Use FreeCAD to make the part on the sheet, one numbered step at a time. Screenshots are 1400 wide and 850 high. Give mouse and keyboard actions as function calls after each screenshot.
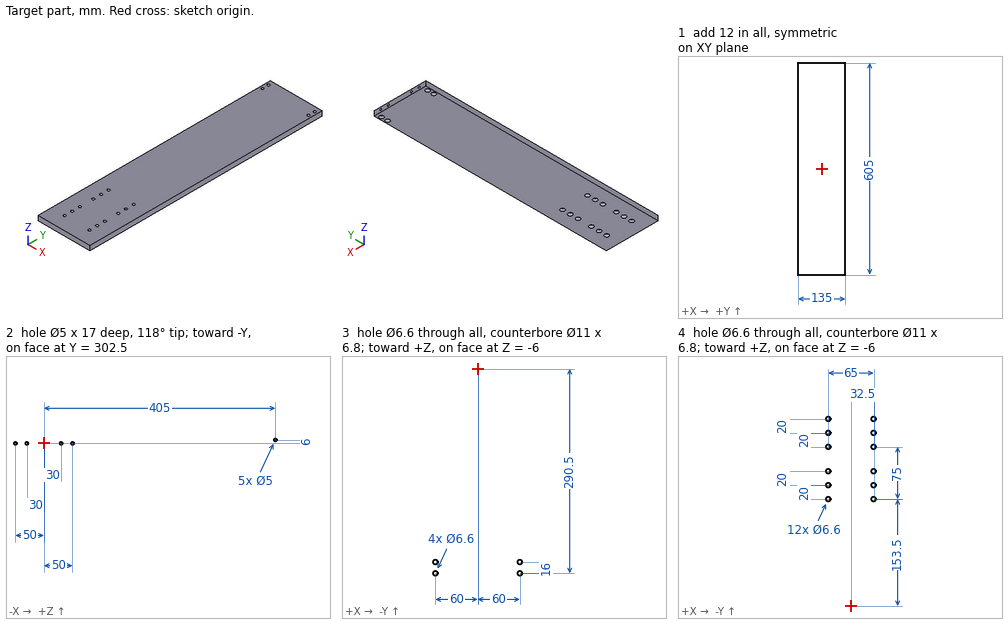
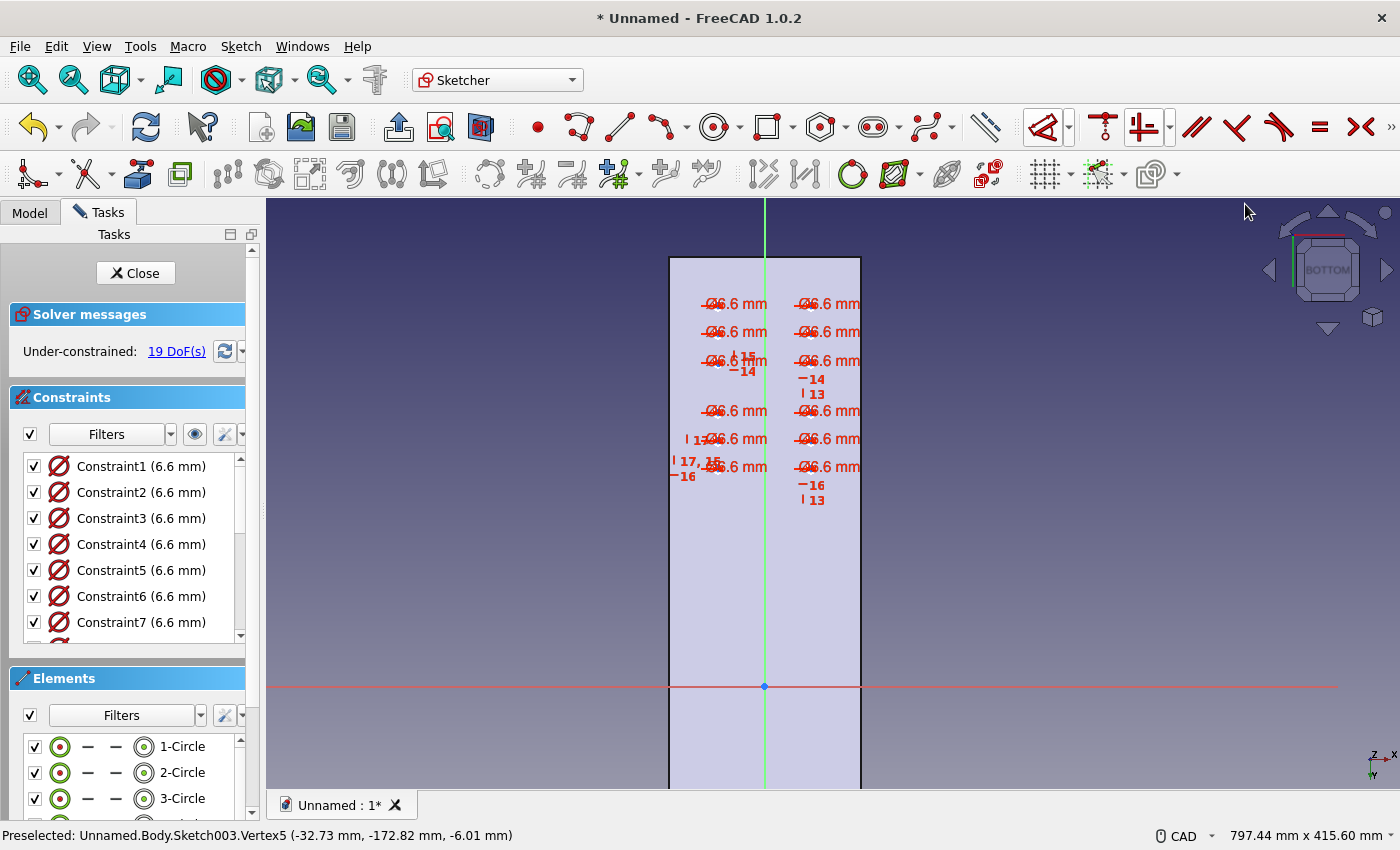
click(718, 363)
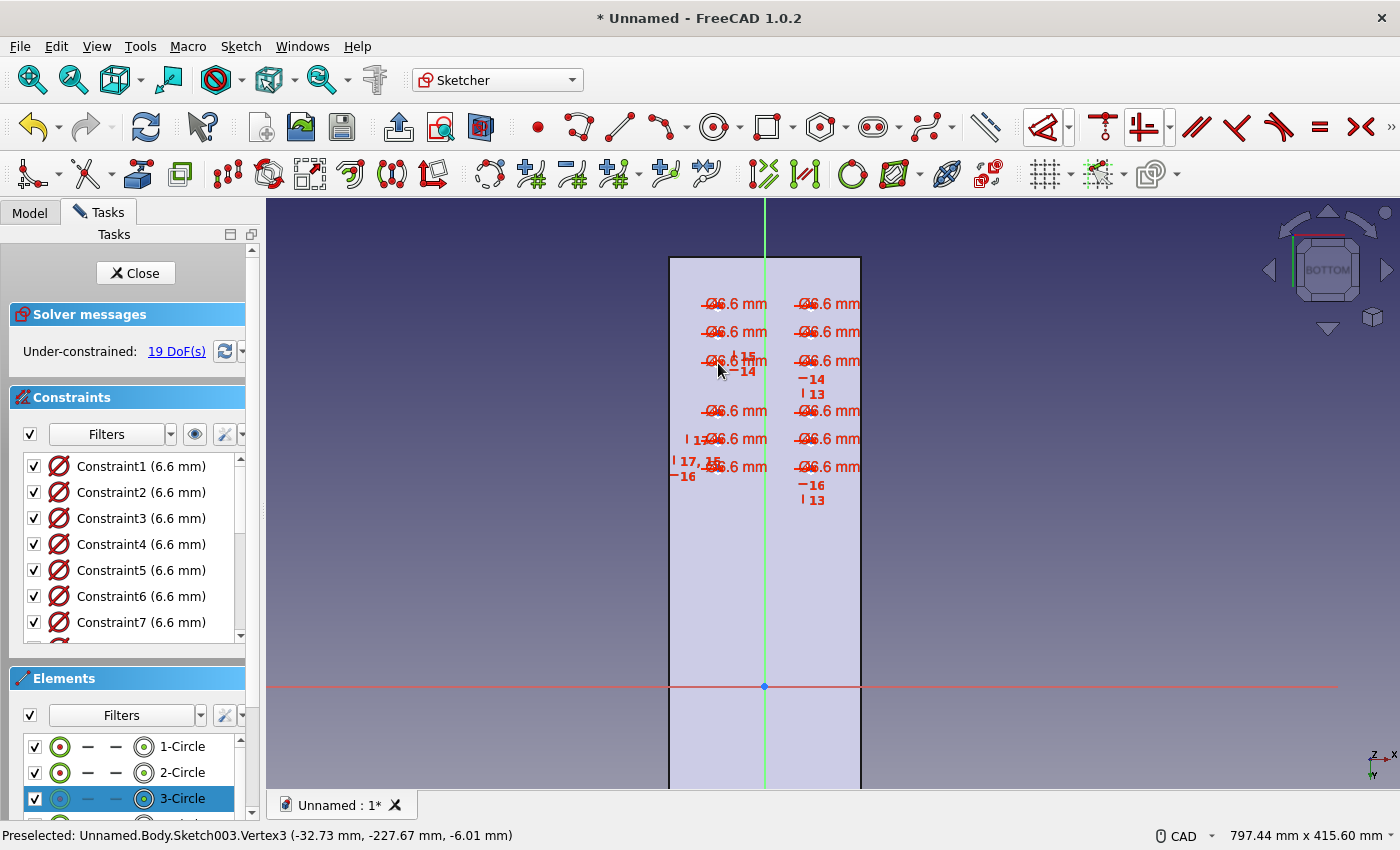
click(718, 334)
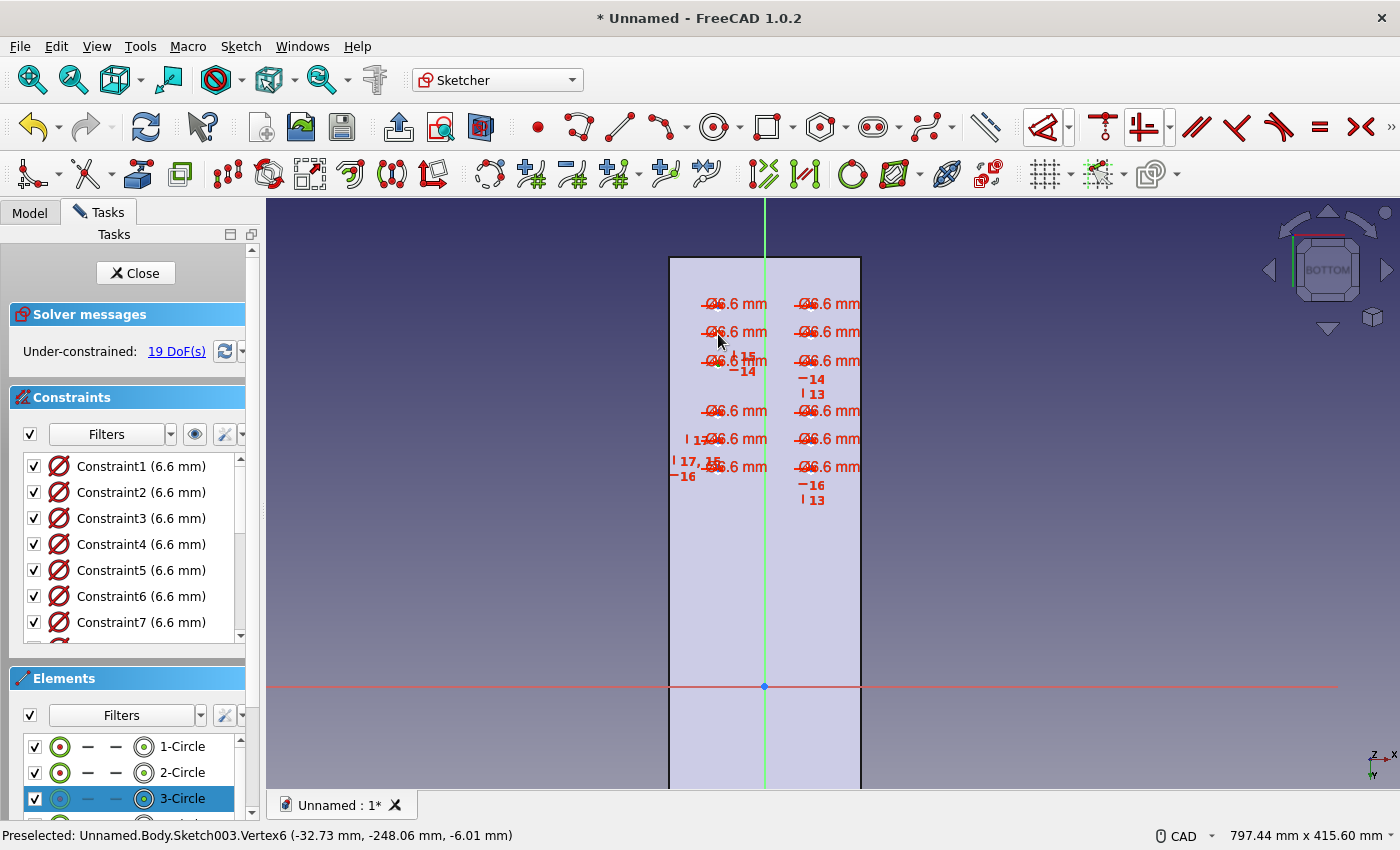
key(v)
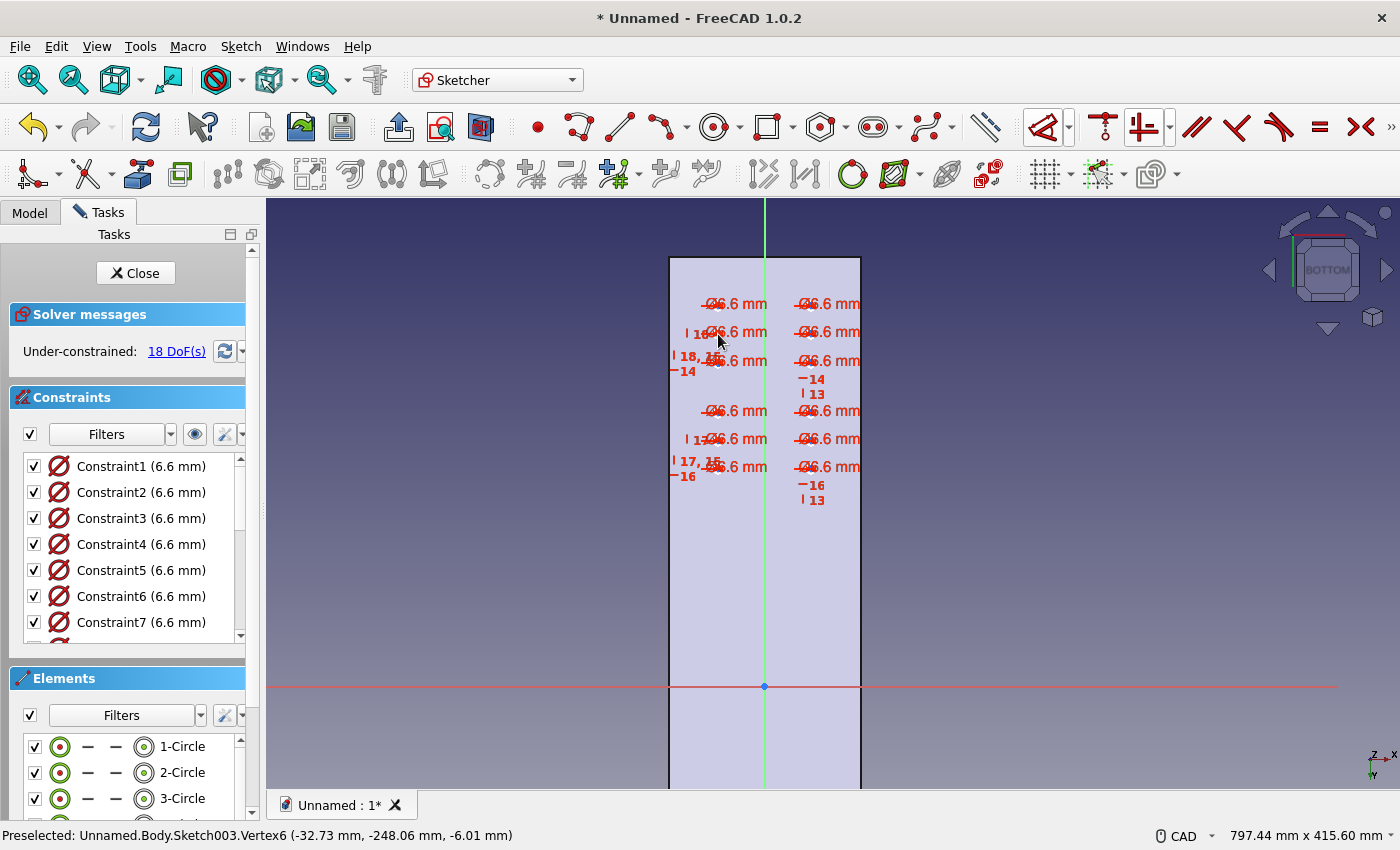
click(811, 363)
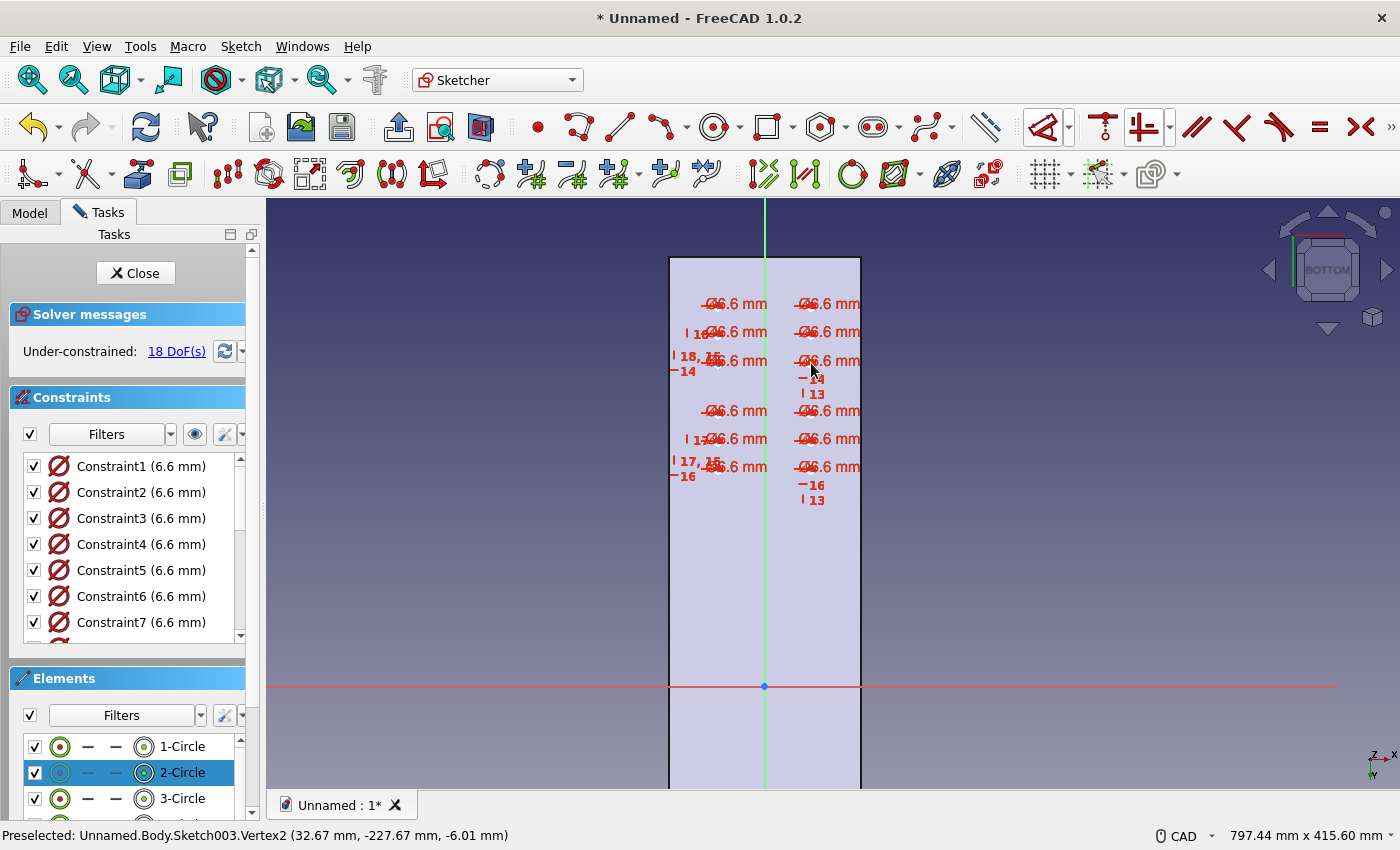
click(811, 334)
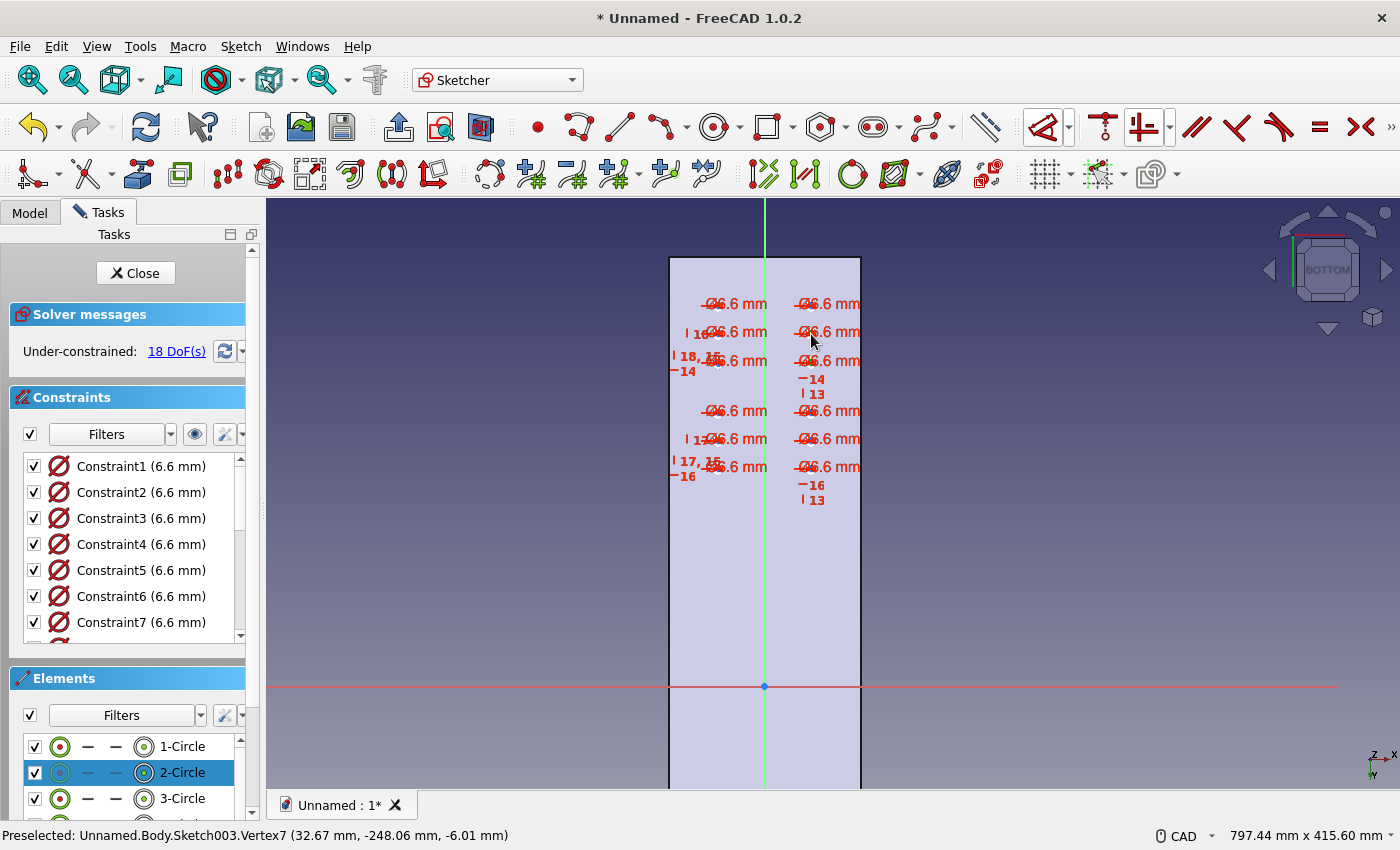
key(v)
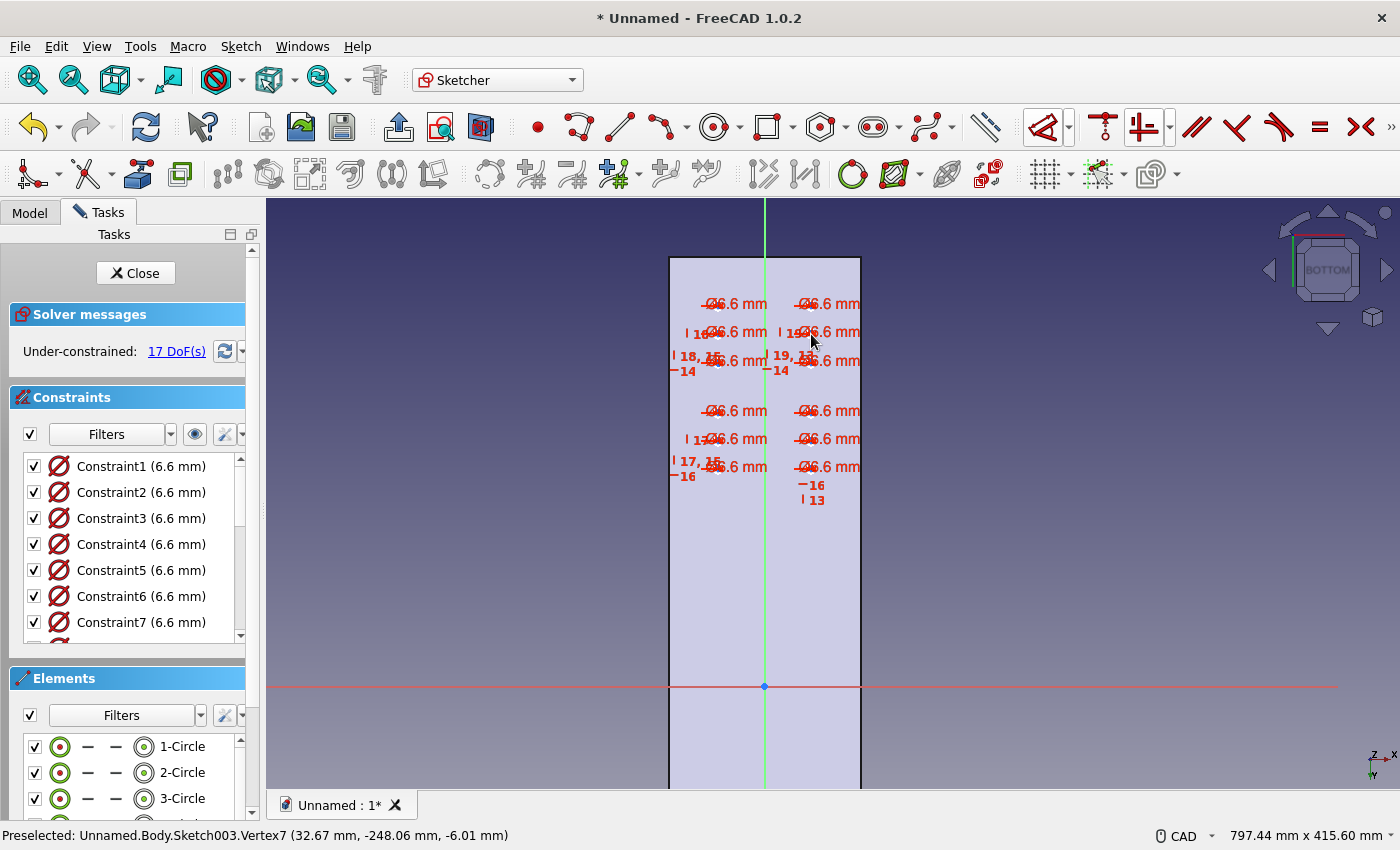
click(718, 334)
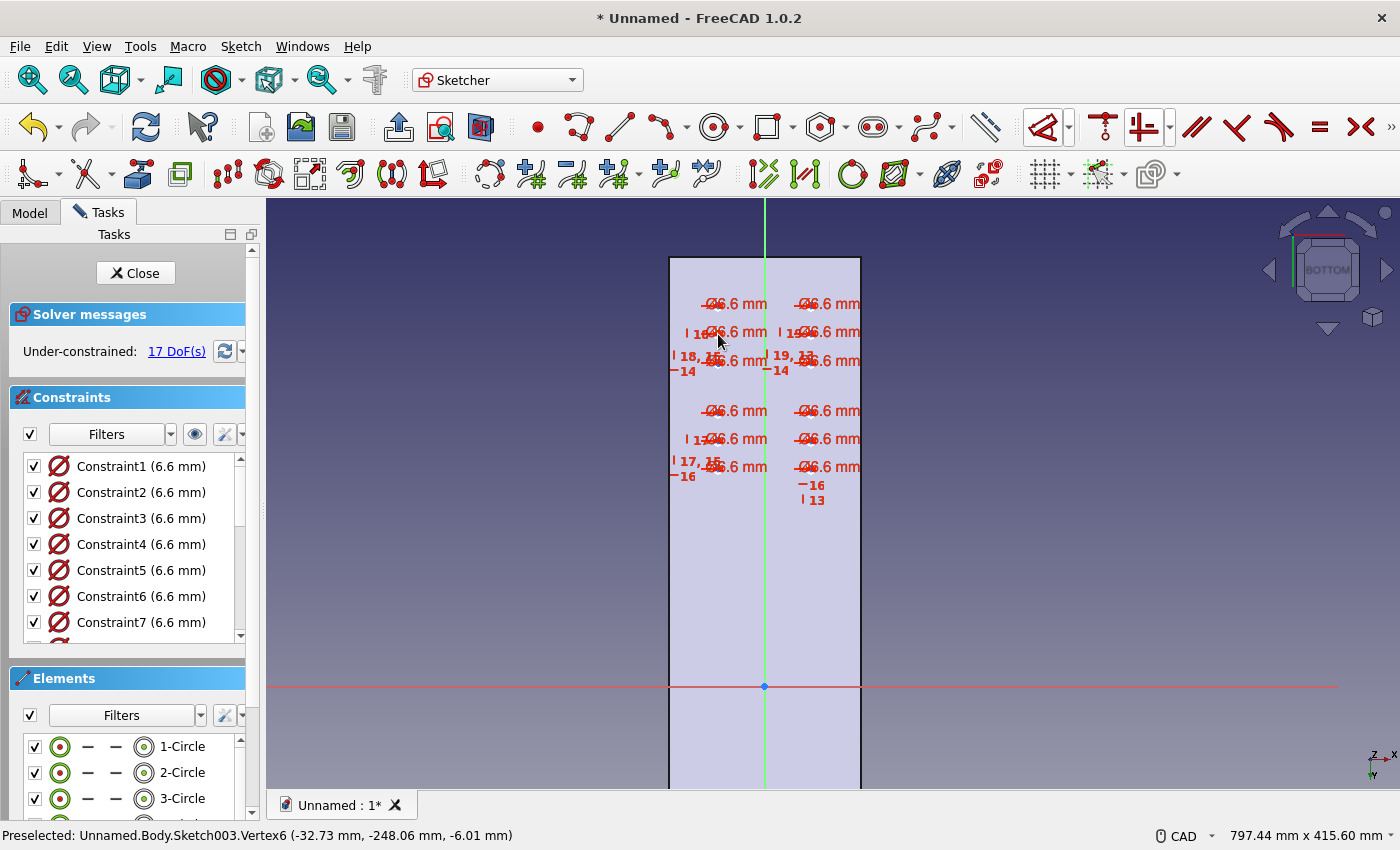
click(811, 334)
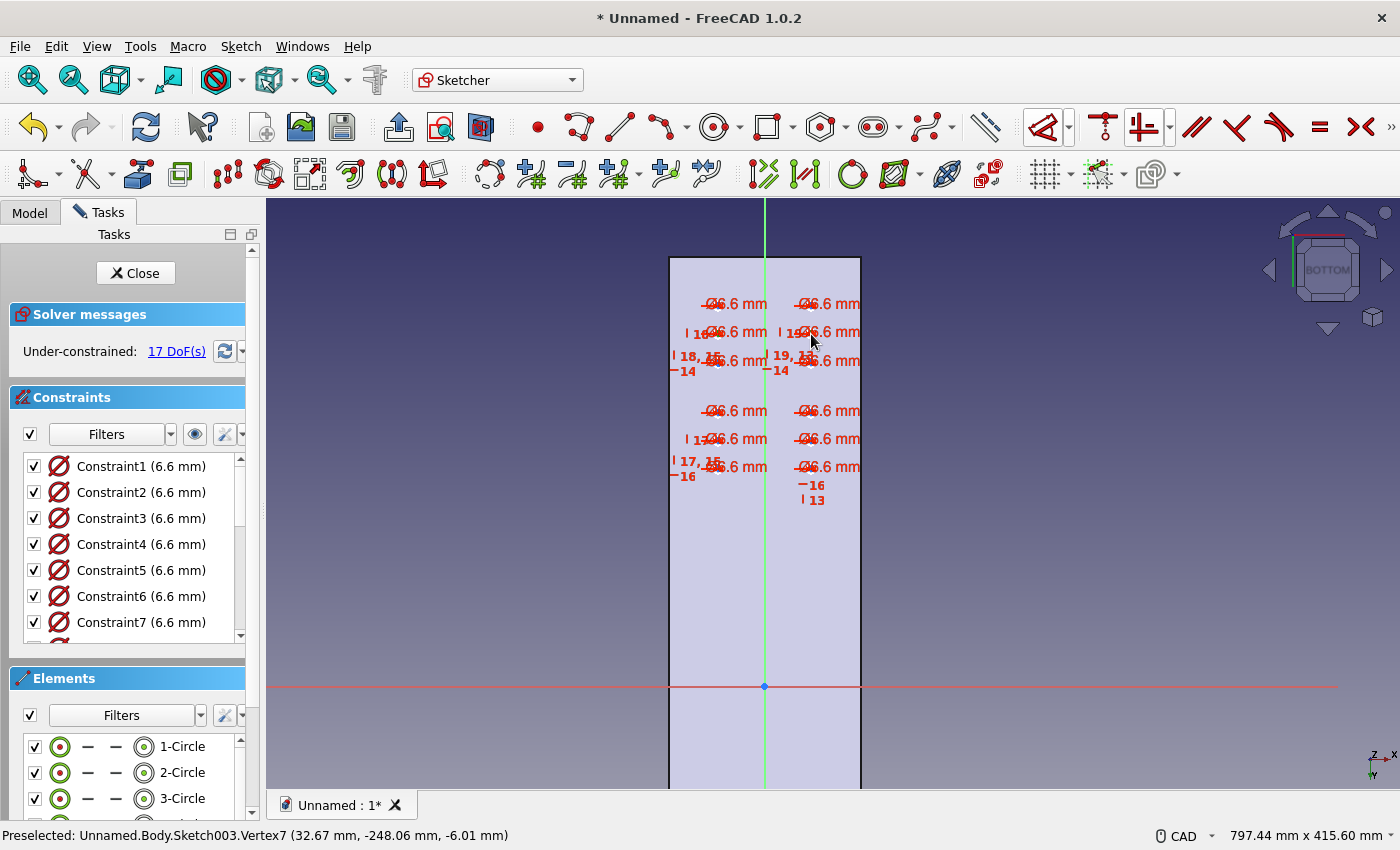
key(h)